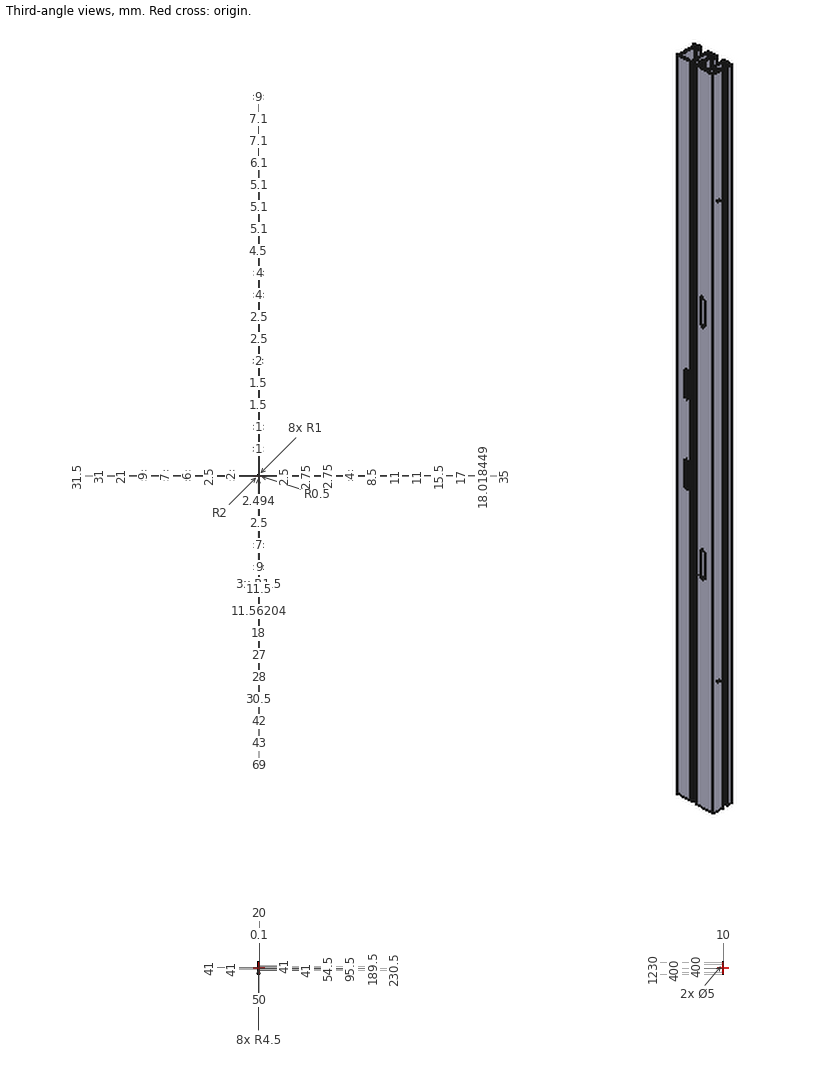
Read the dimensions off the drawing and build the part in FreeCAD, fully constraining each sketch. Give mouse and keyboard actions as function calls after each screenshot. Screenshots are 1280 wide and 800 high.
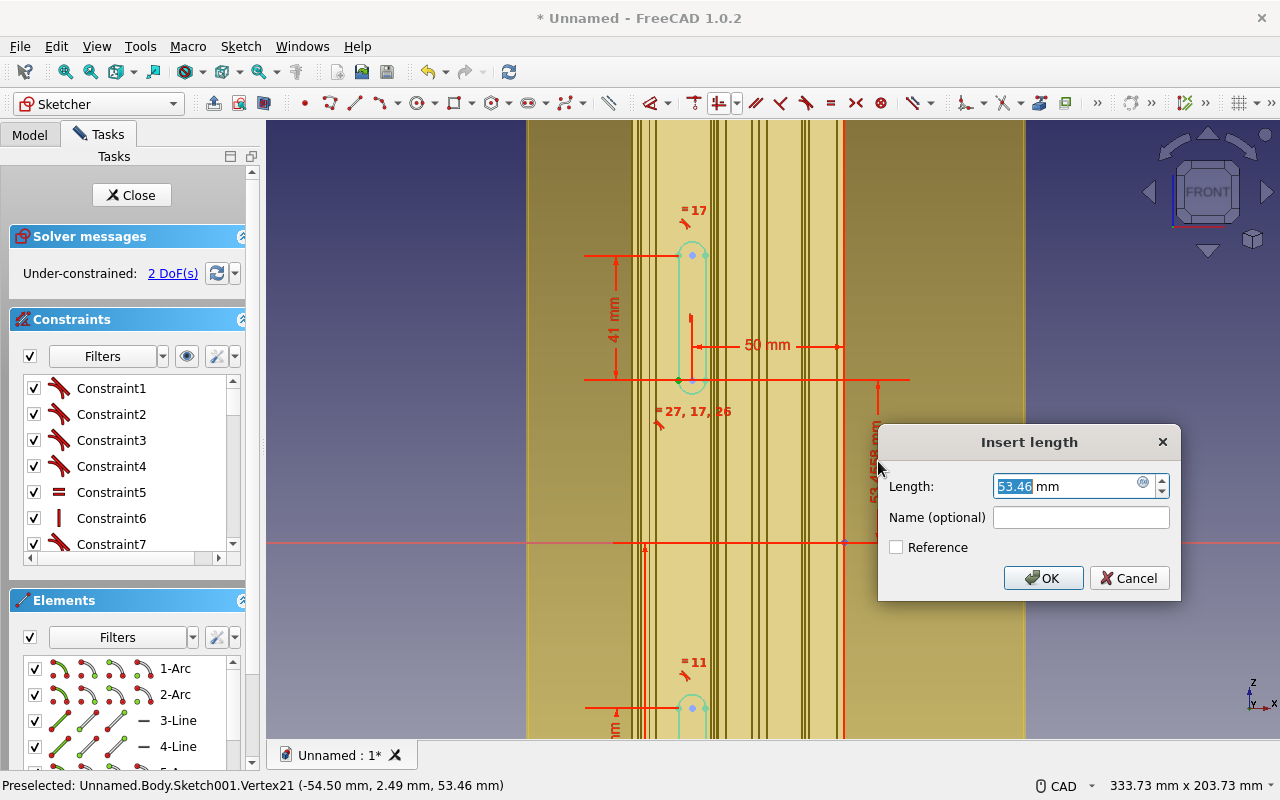
text(54.5)
key(Return)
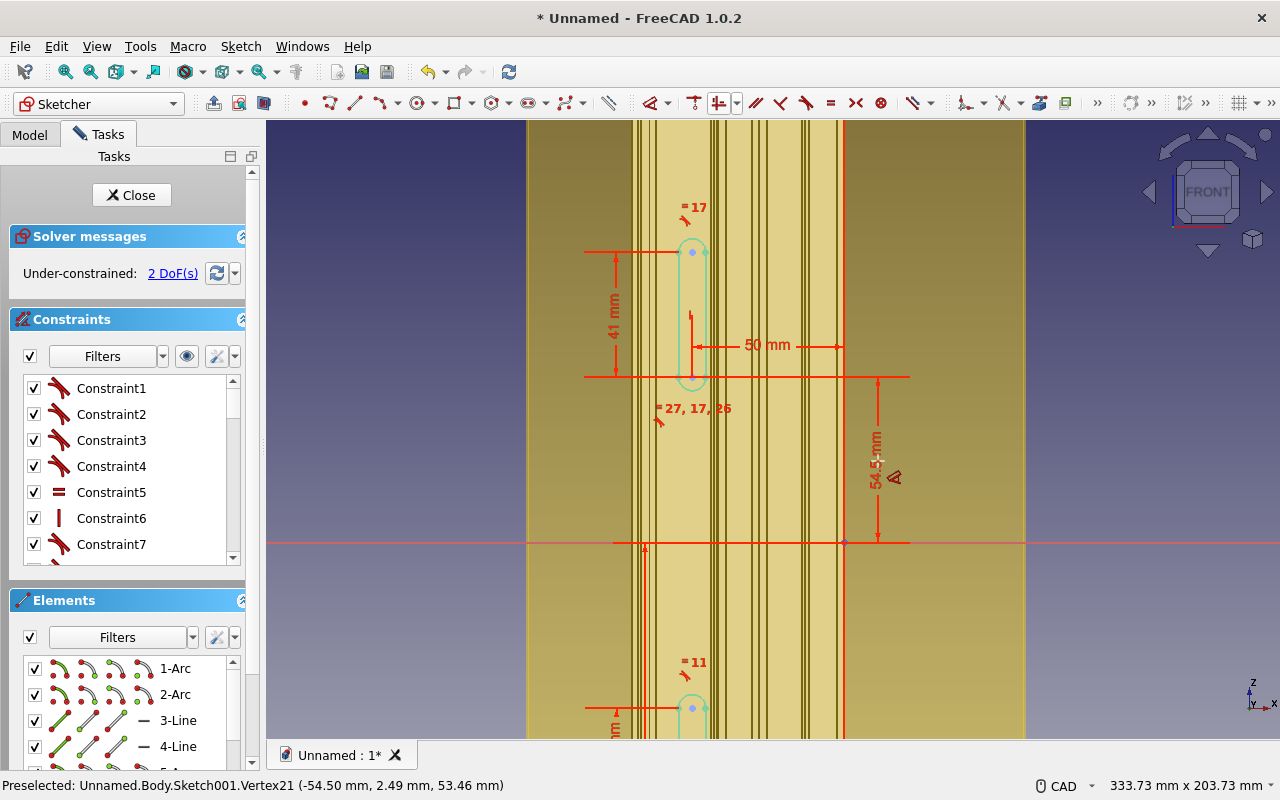
scroll(680, 381, down, 6)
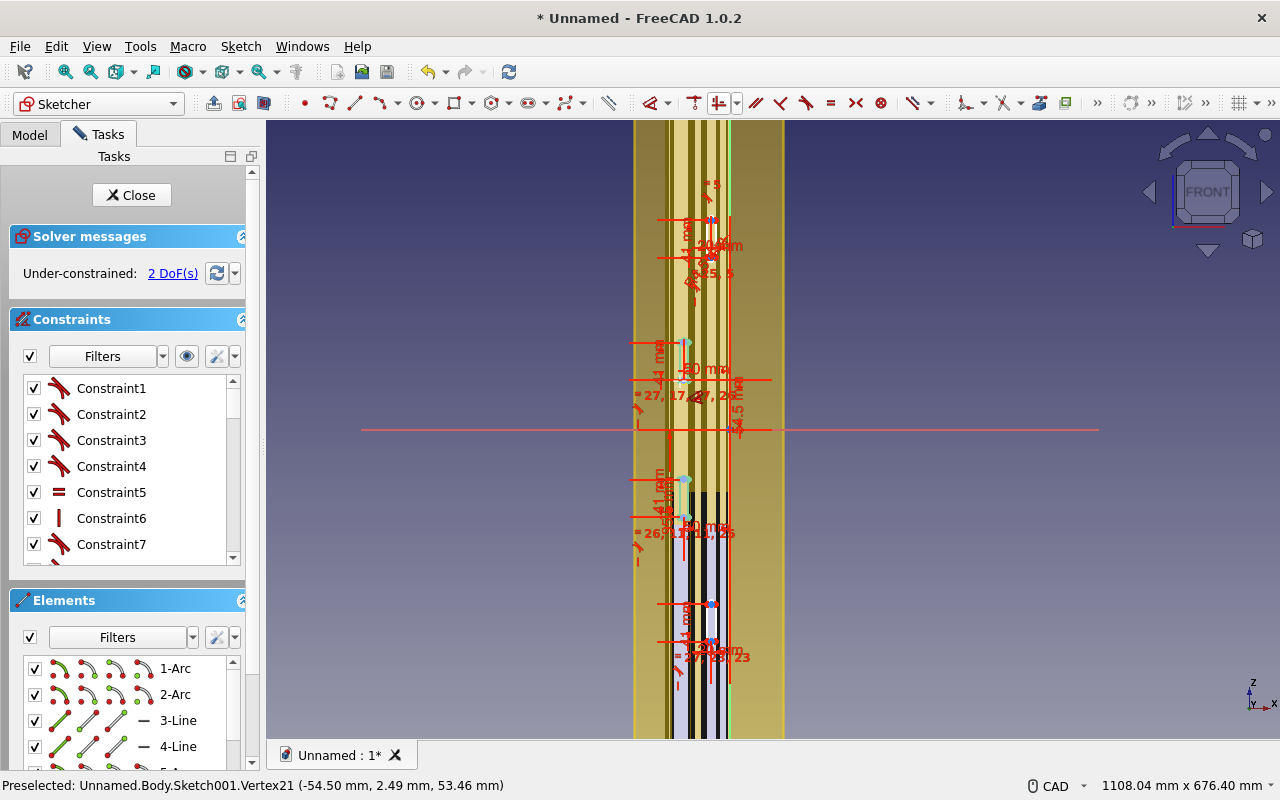
scroll(707, 258, up, 6)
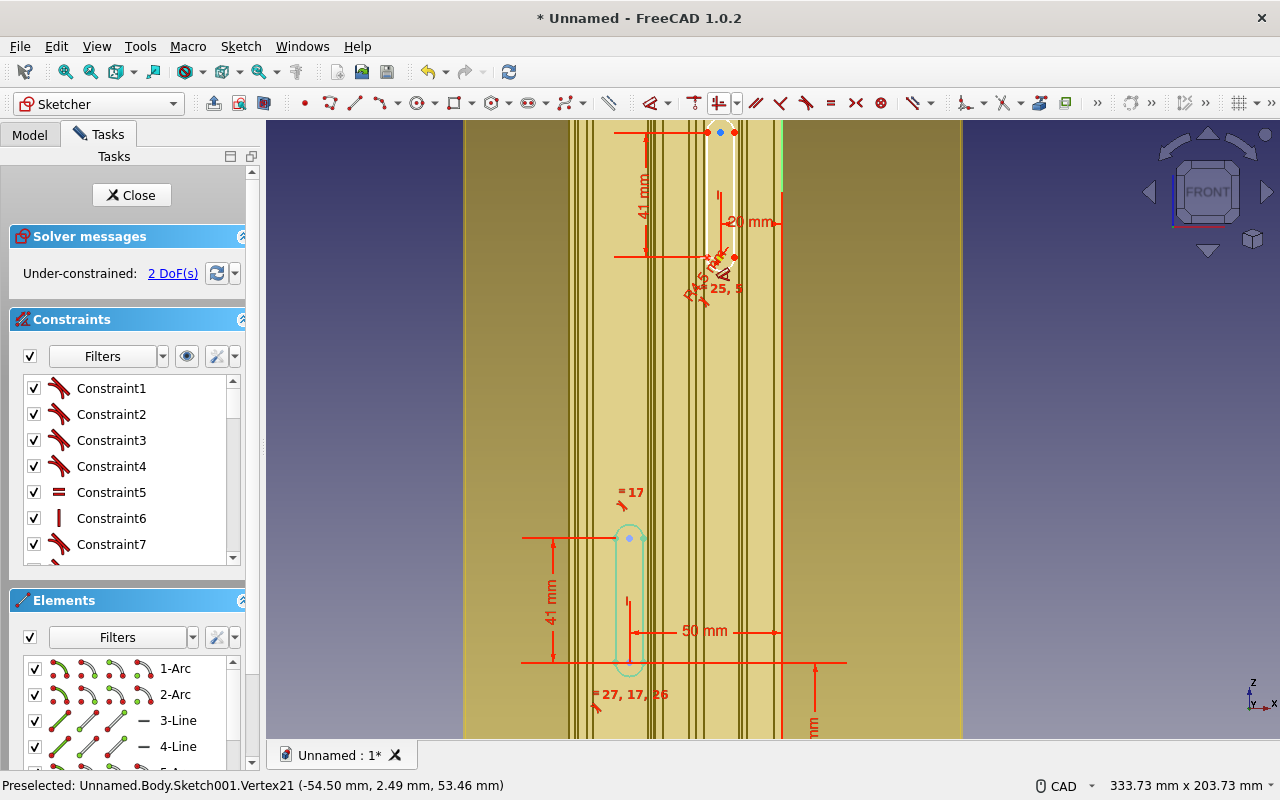
click(707, 257)
click(816, 484)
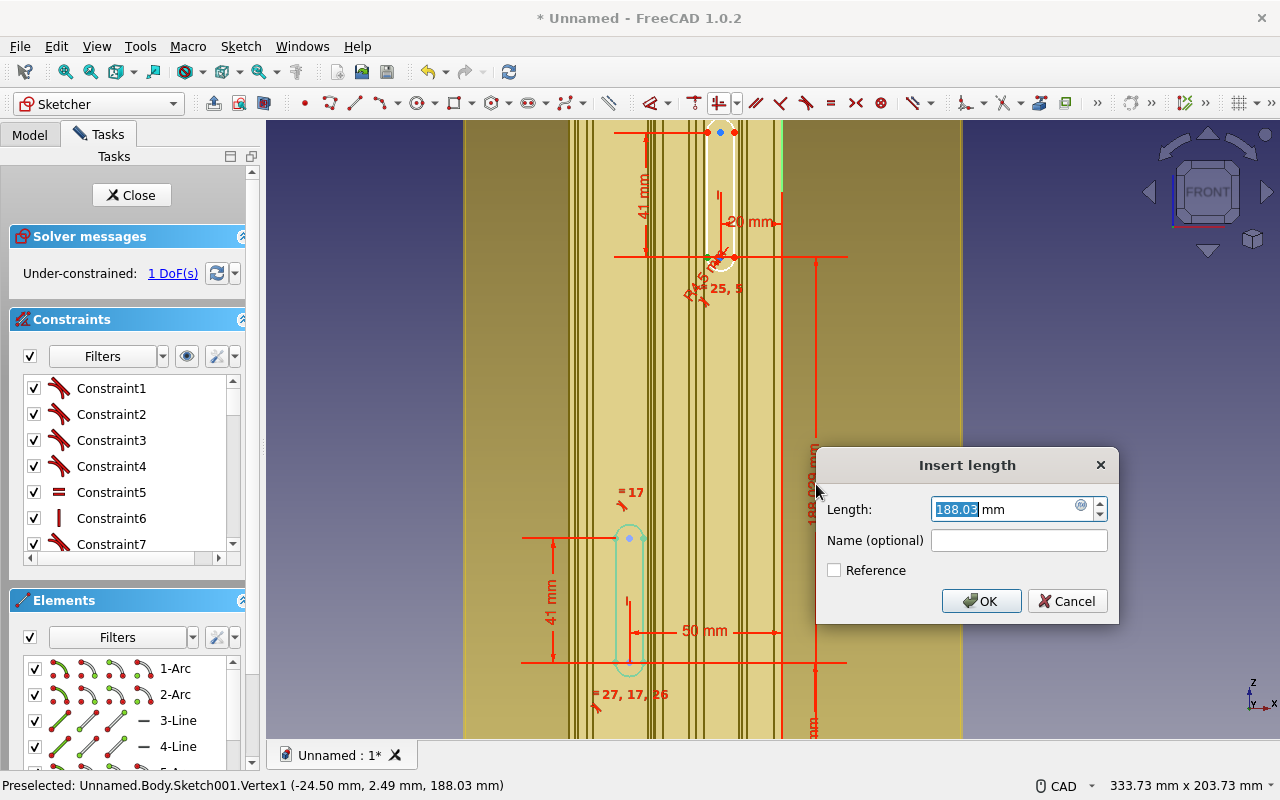
text(189.5)
key(Return)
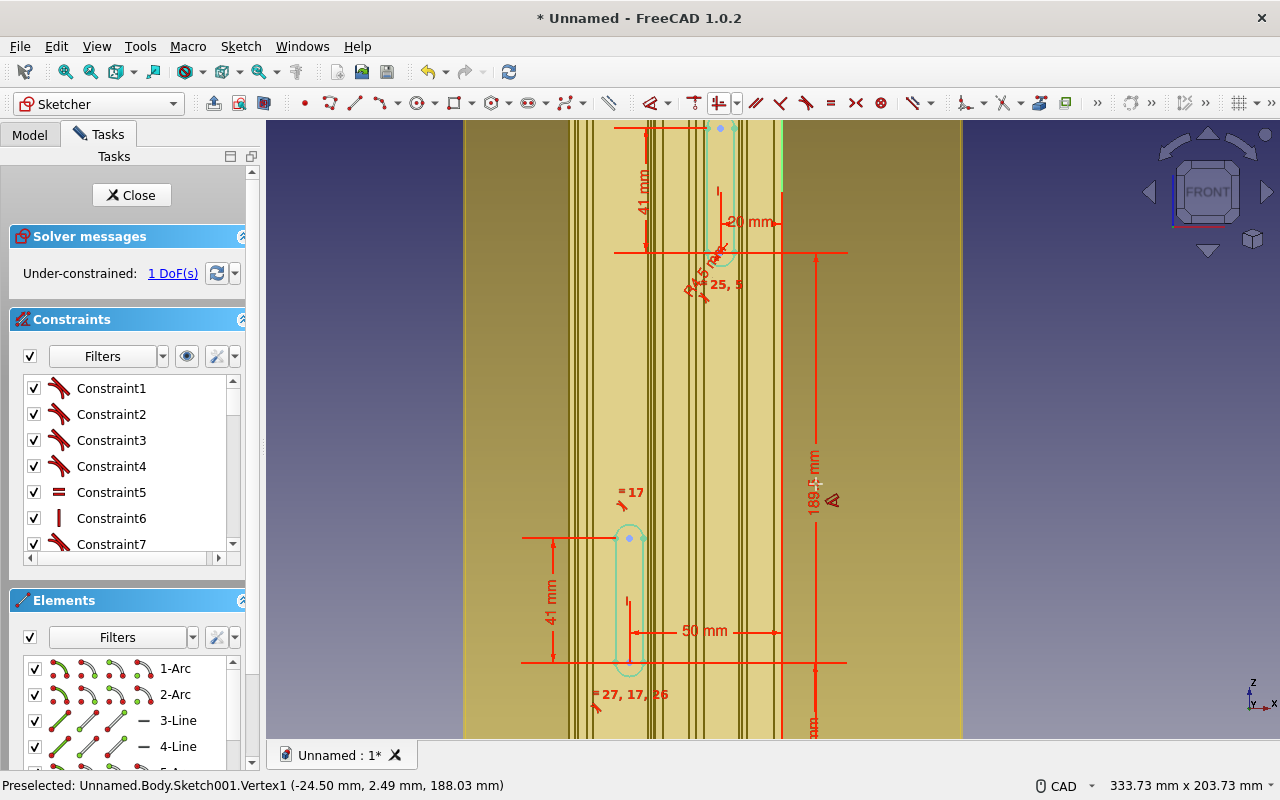
scroll(707, 258, down, 6)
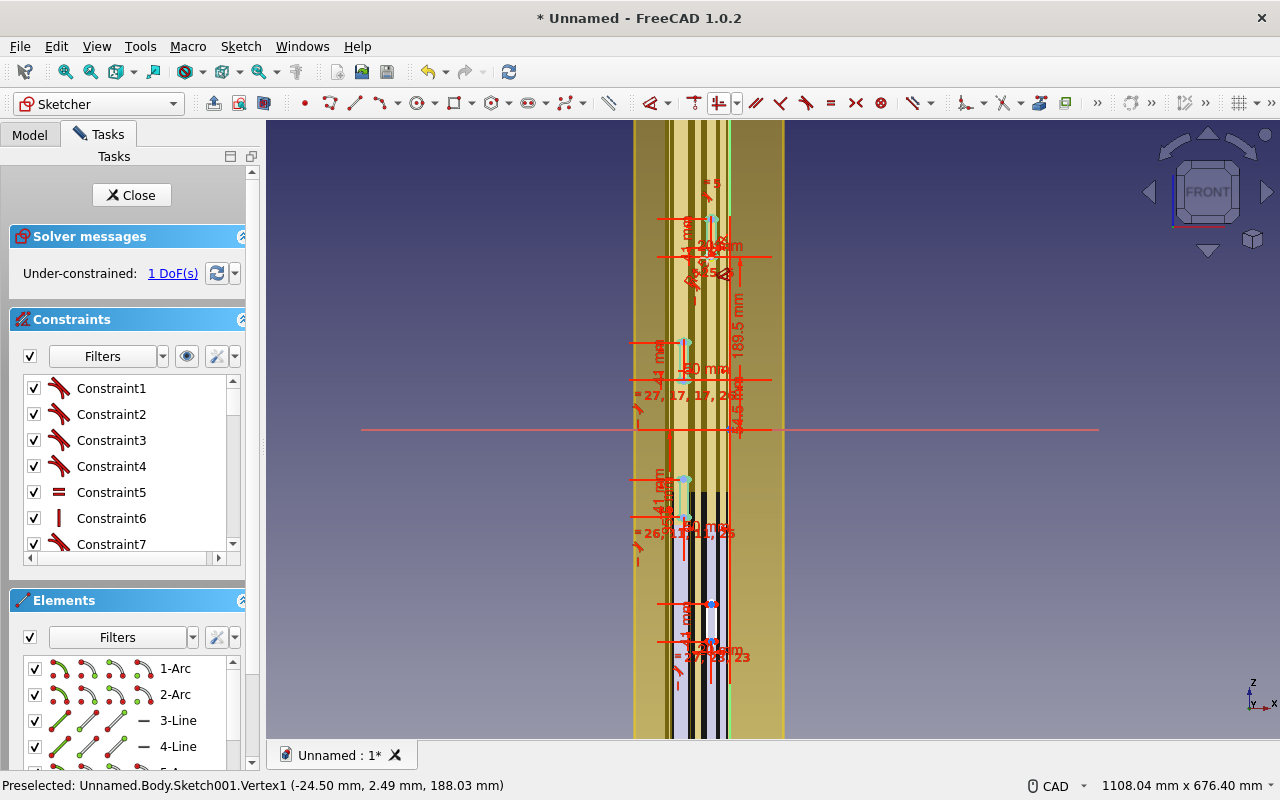
scroll(707, 642, up, 6)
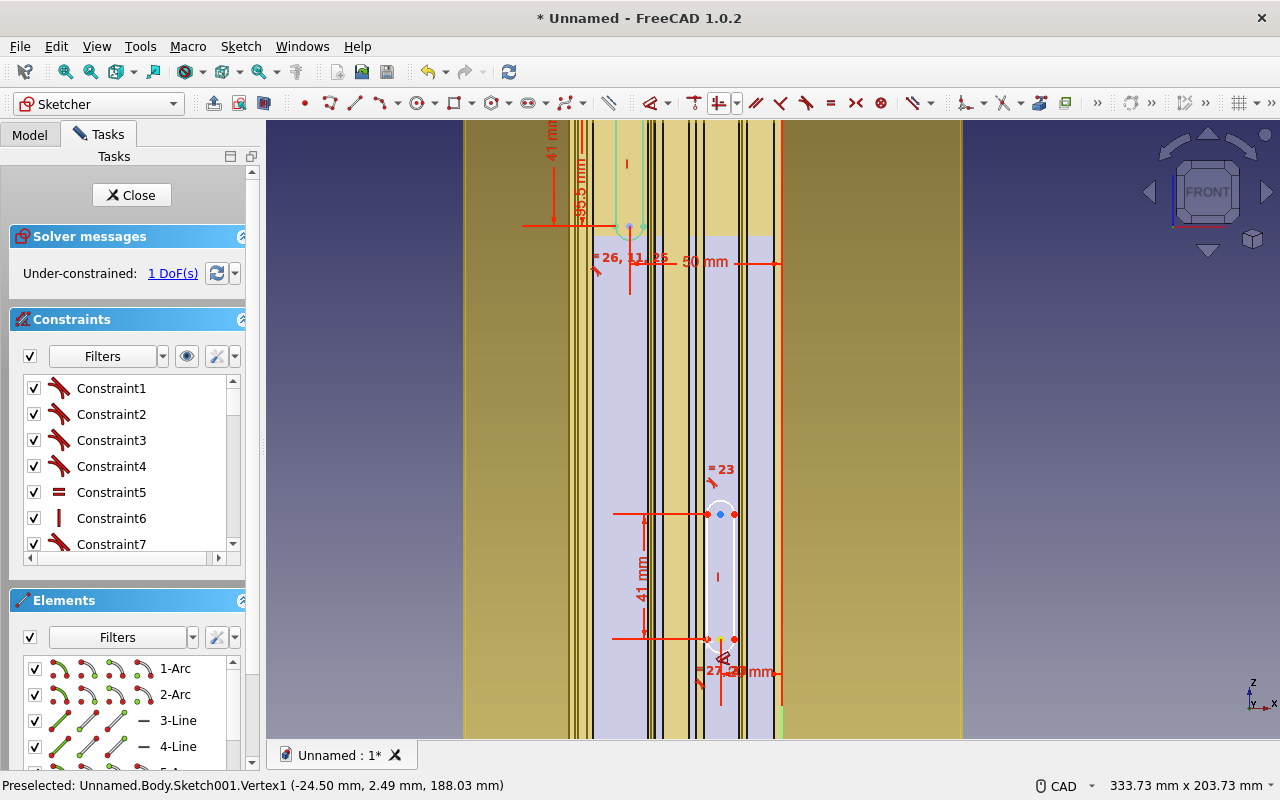
click(707, 639)
click(816, 394)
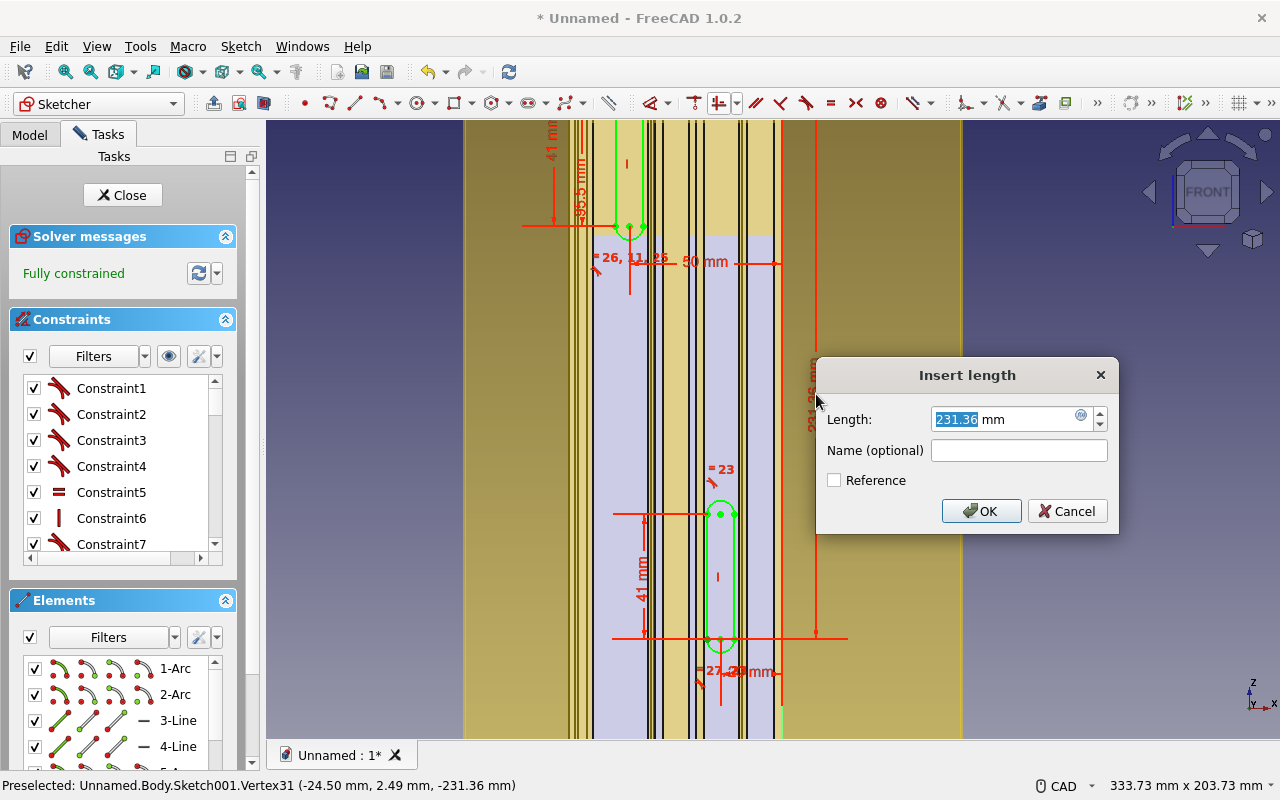
text(230.5)
key(Return)
key(Escape)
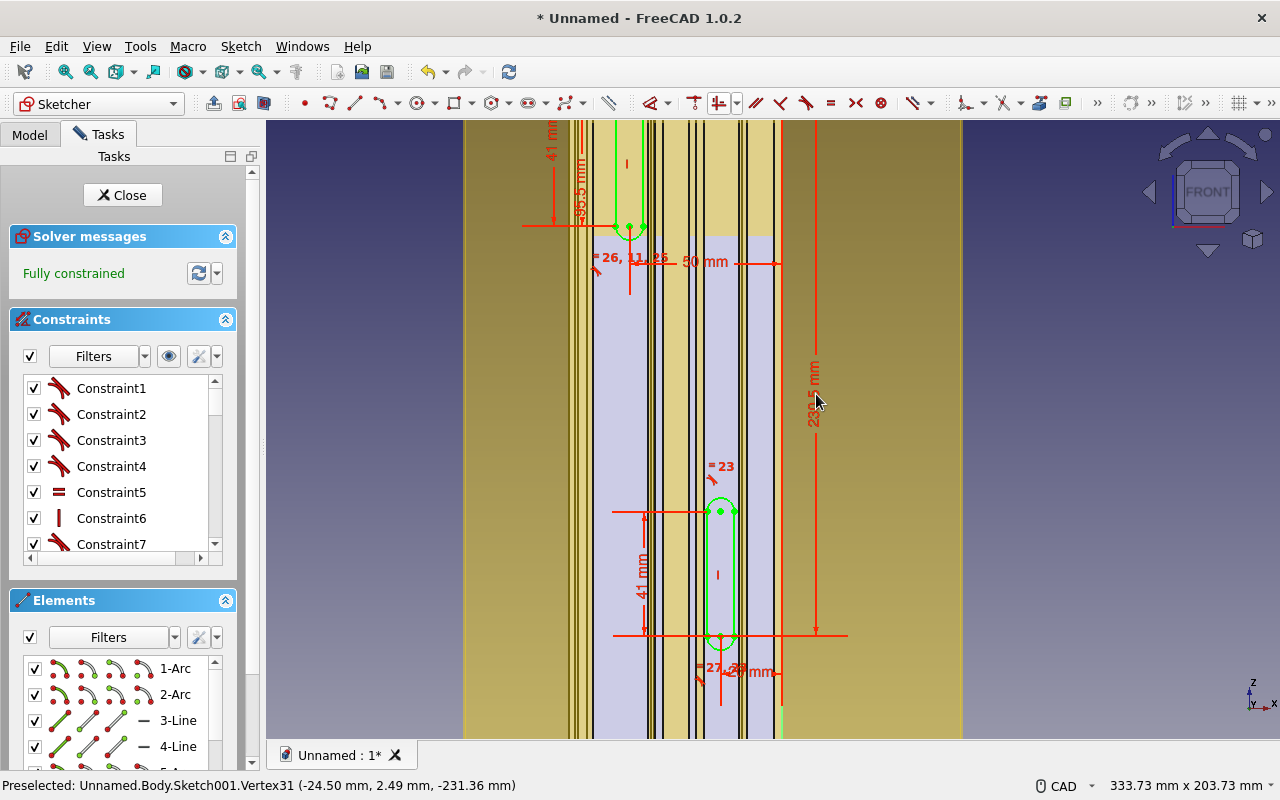
click(123, 195)